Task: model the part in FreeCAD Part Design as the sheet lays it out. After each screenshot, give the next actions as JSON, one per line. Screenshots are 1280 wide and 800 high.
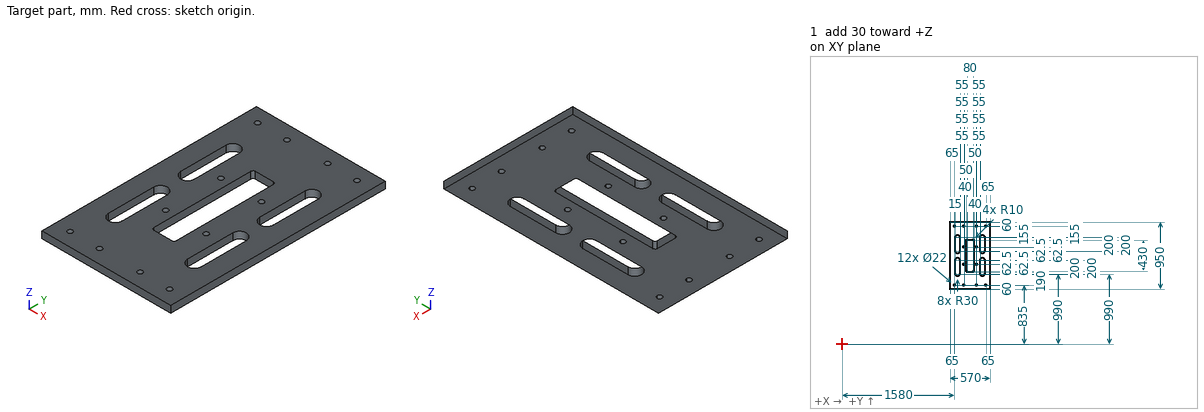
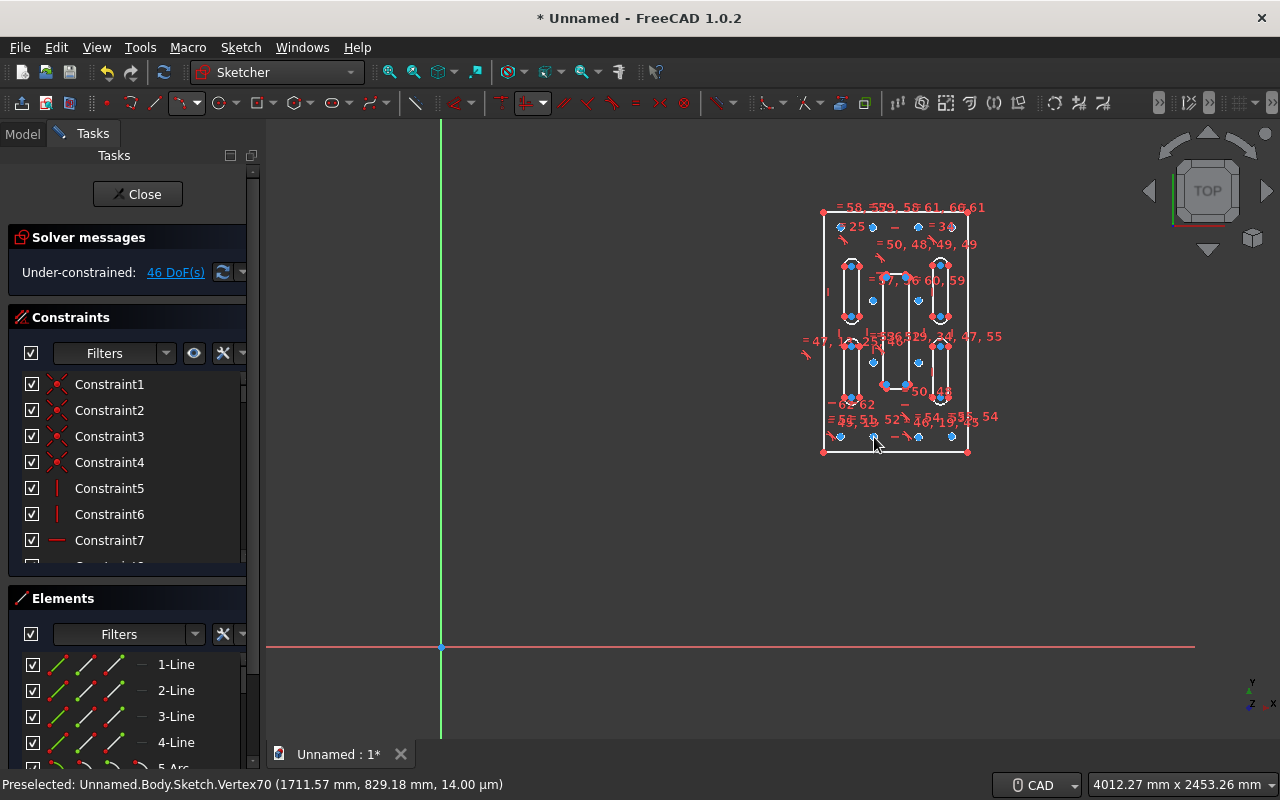
{"action": "left_click", "coordinate": [874, 437]}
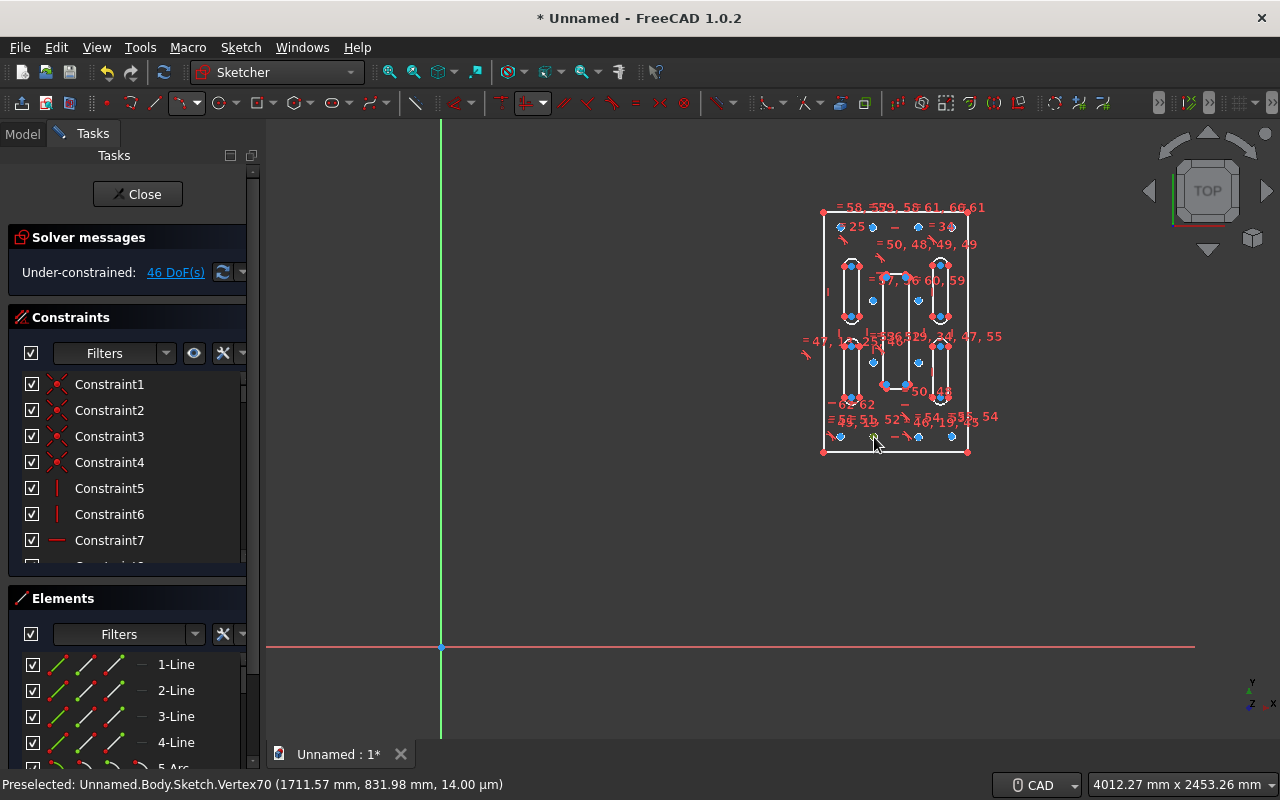
{"action": "left_click", "coordinate": [919, 437]}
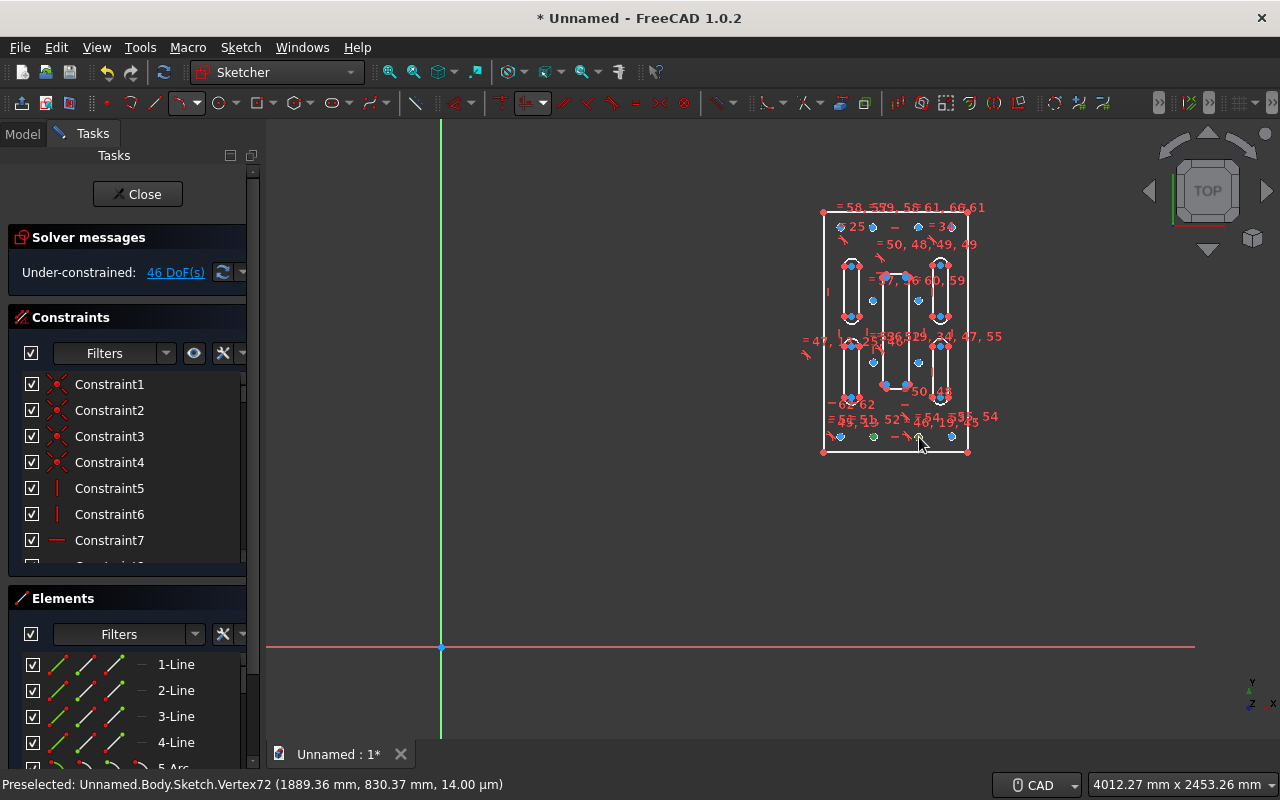
{"action": "left_click", "coordinate": [546, 104]}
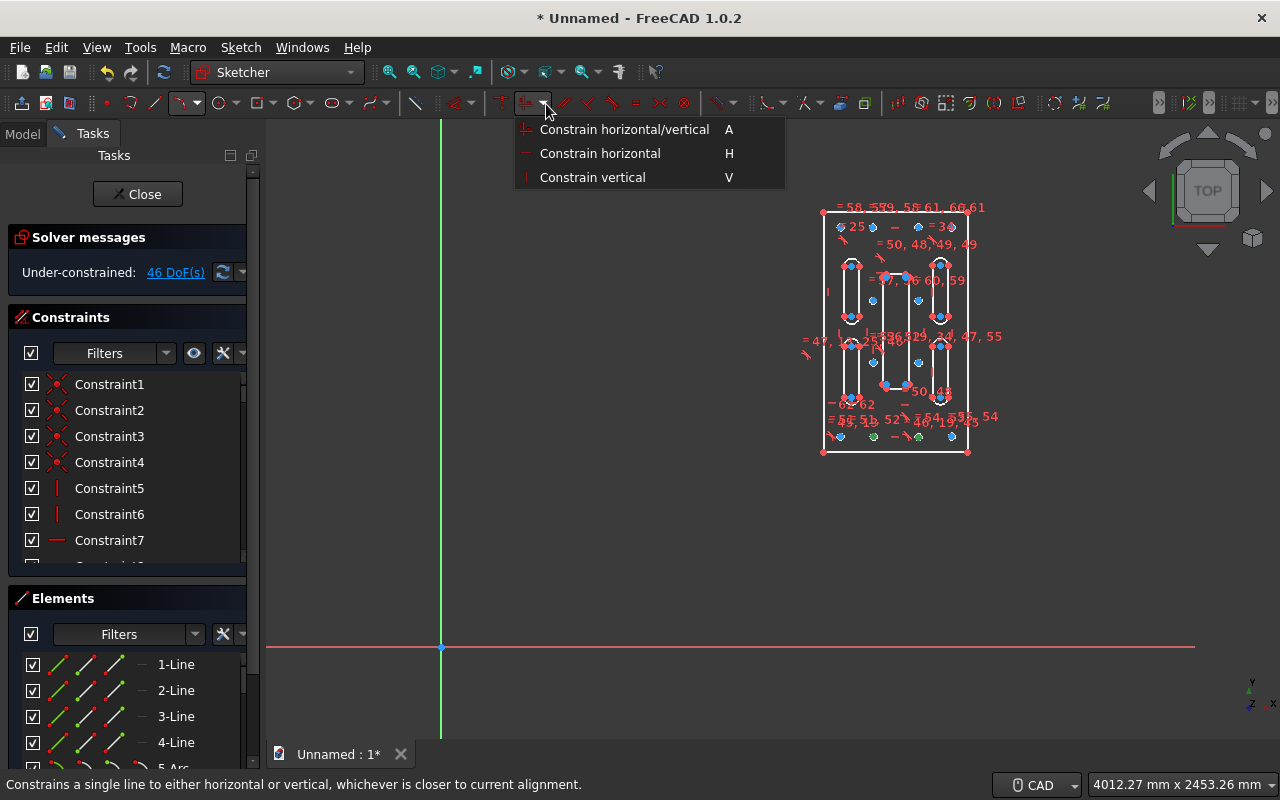
{"action": "left_click", "coordinate": [650, 153]}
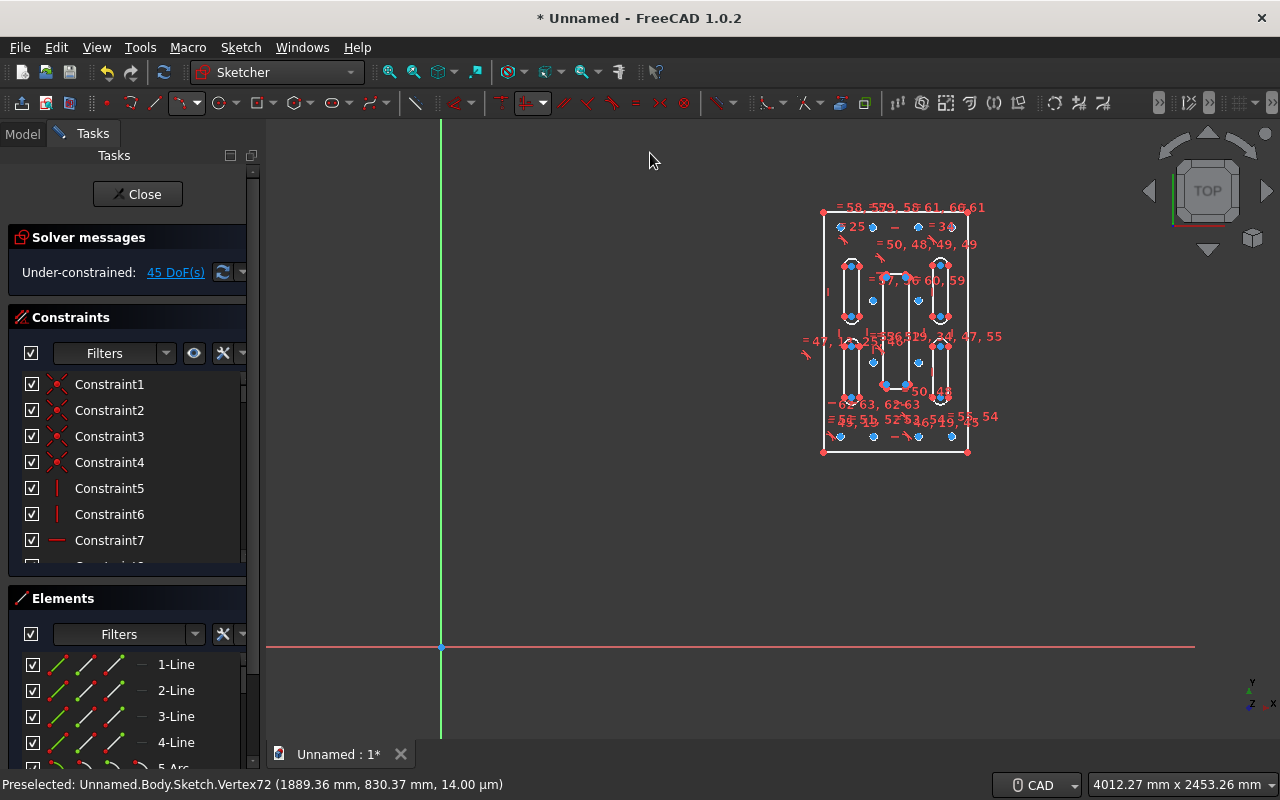
{"action": "left_click", "coordinate": [919, 437]}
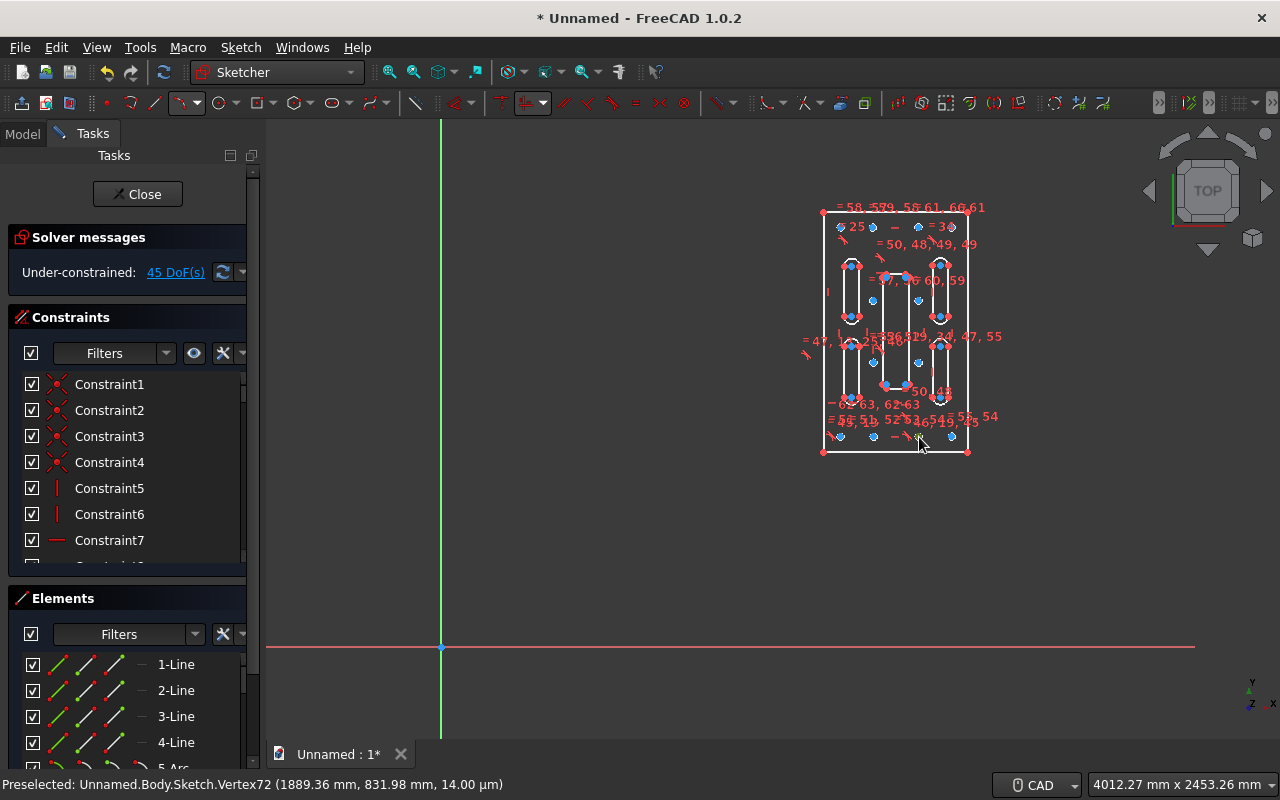
{"action": "left_click", "coordinate": [952, 437]}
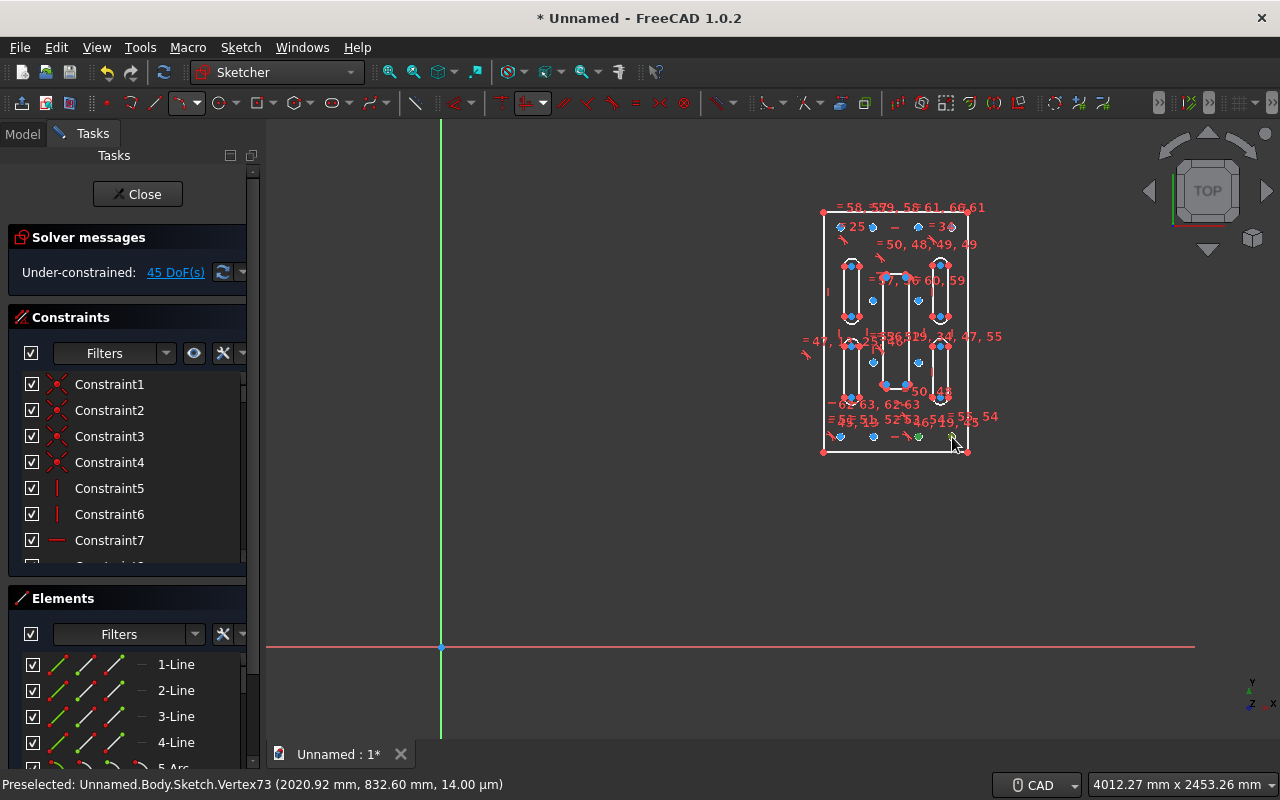
{"action": "left_click", "coordinate": [546, 104]}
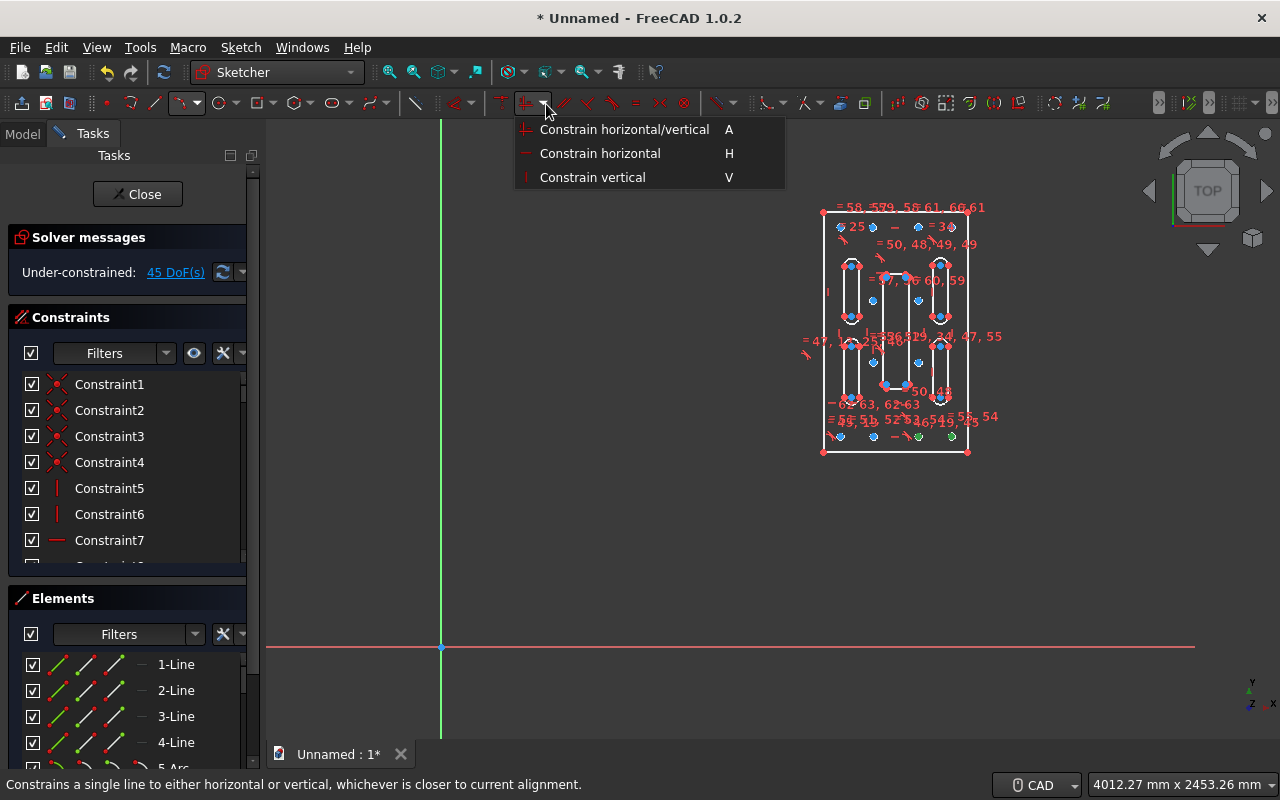
{"action": "left_click", "coordinate": [650, 153]}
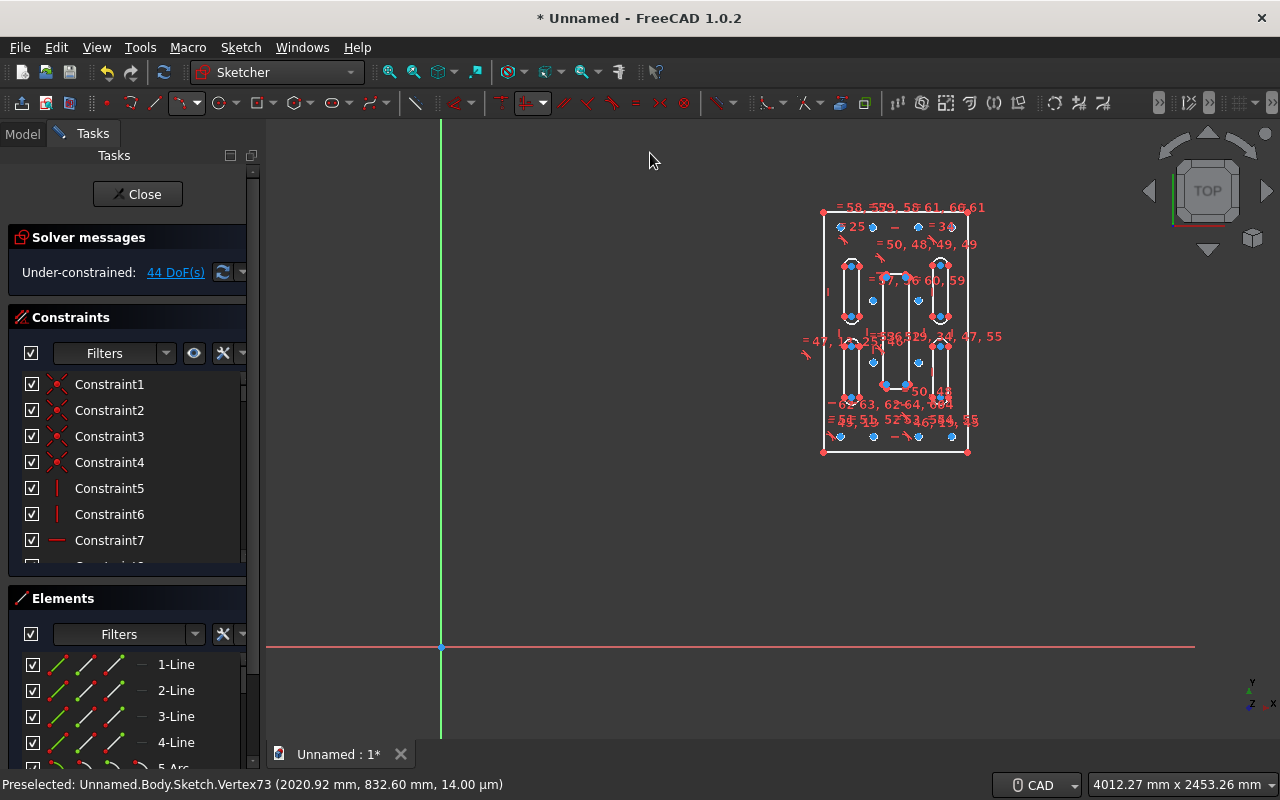
{"action": "scroll", "coordinate": [841, 227], "scroll_direction": "up", "scroll_amount": 4}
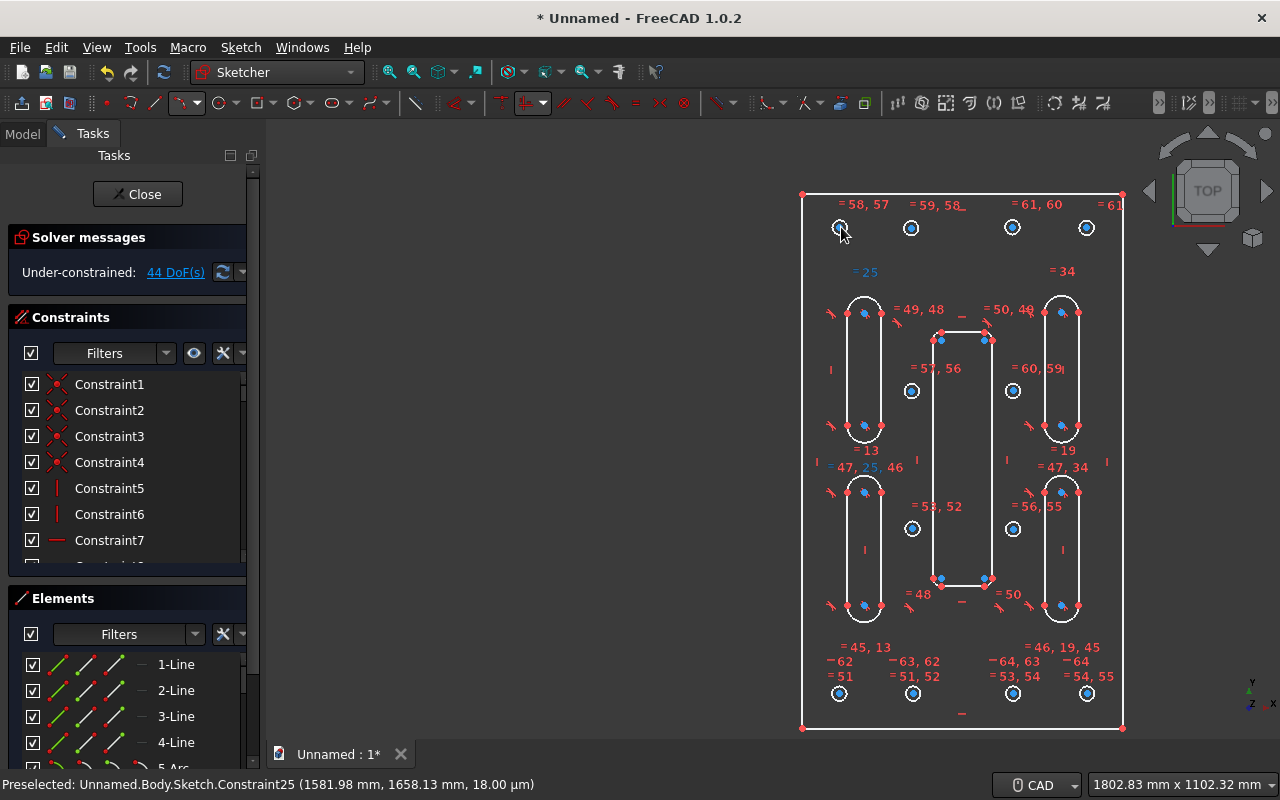
{"action": "left_click", "coordinate": [840, 228]}